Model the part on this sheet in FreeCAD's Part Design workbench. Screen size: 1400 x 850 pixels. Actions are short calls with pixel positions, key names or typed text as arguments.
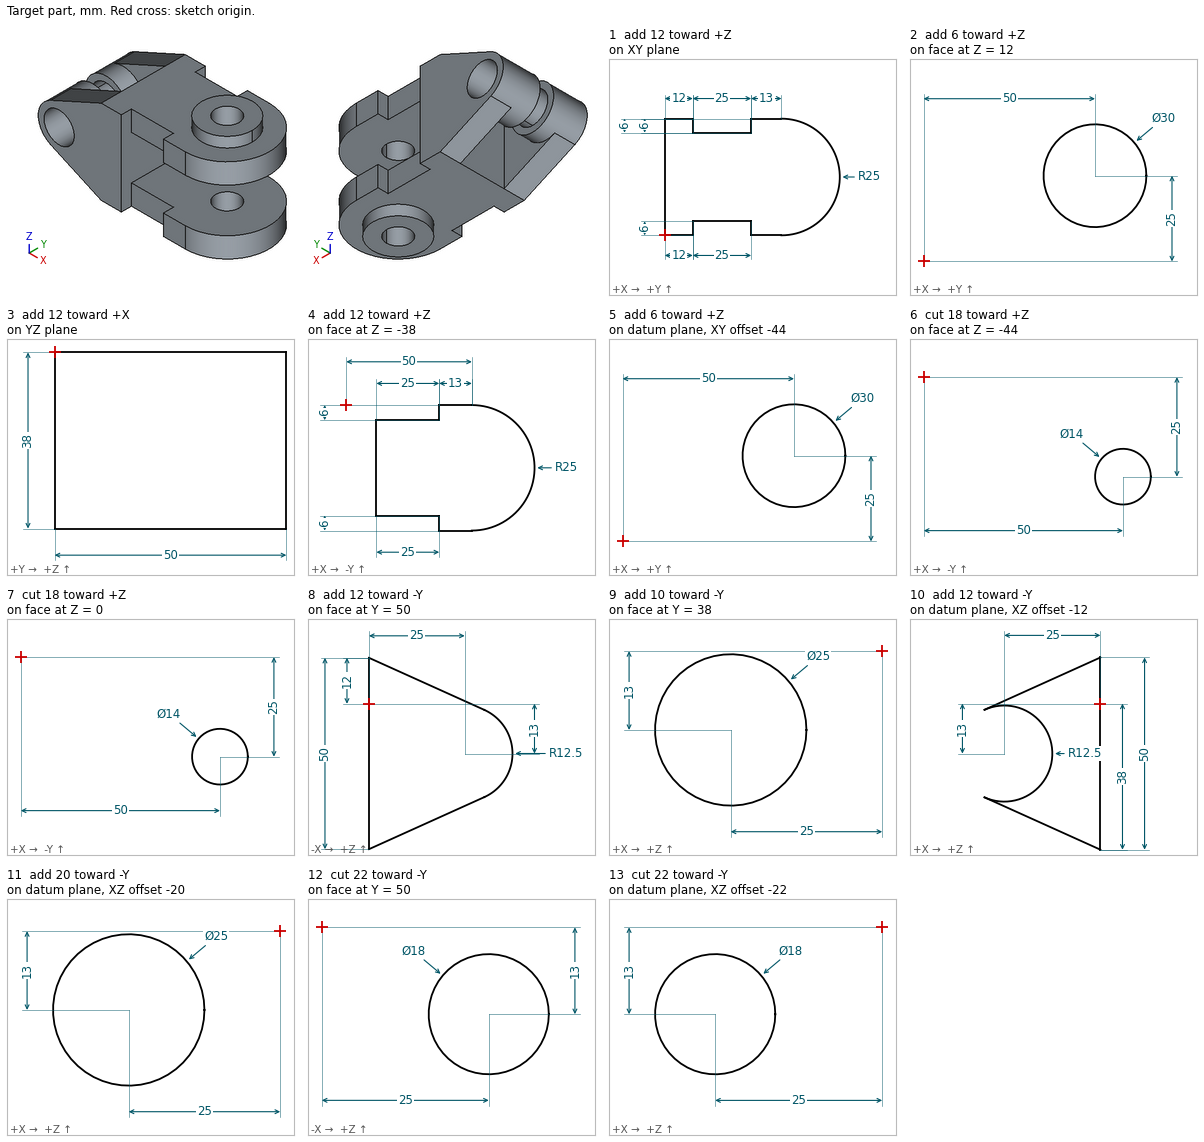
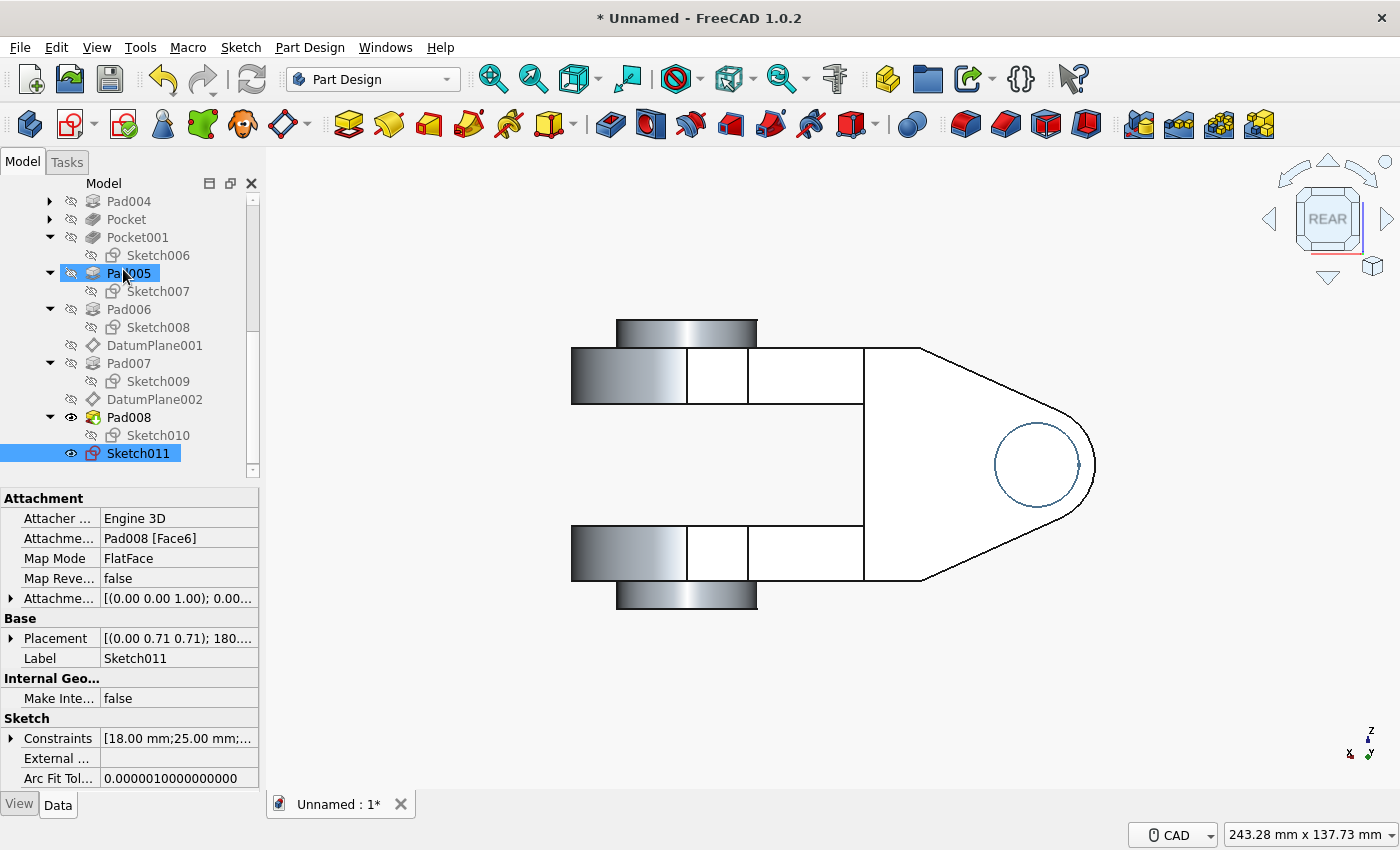
click(612, 124)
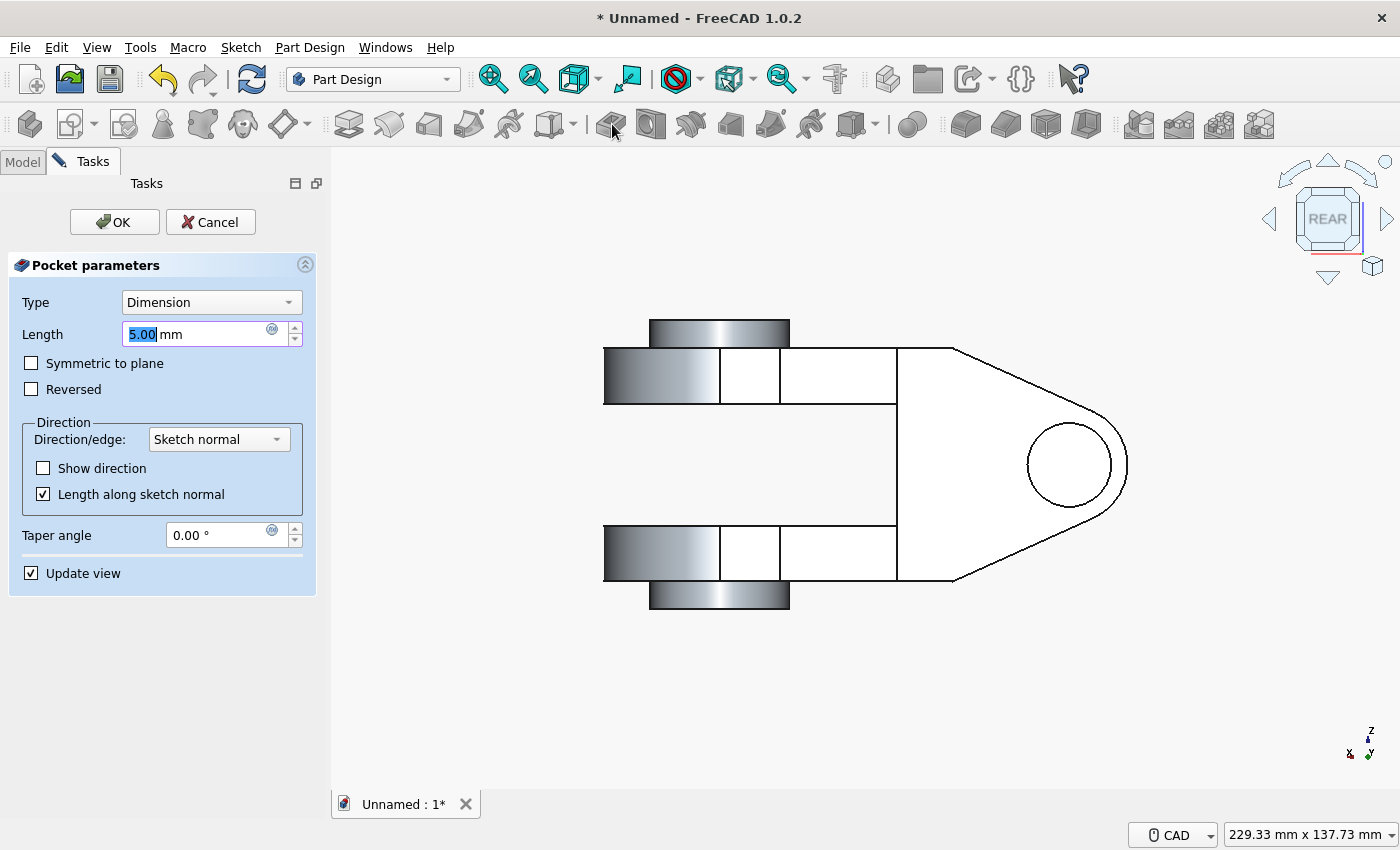
text(22)
key(Tab)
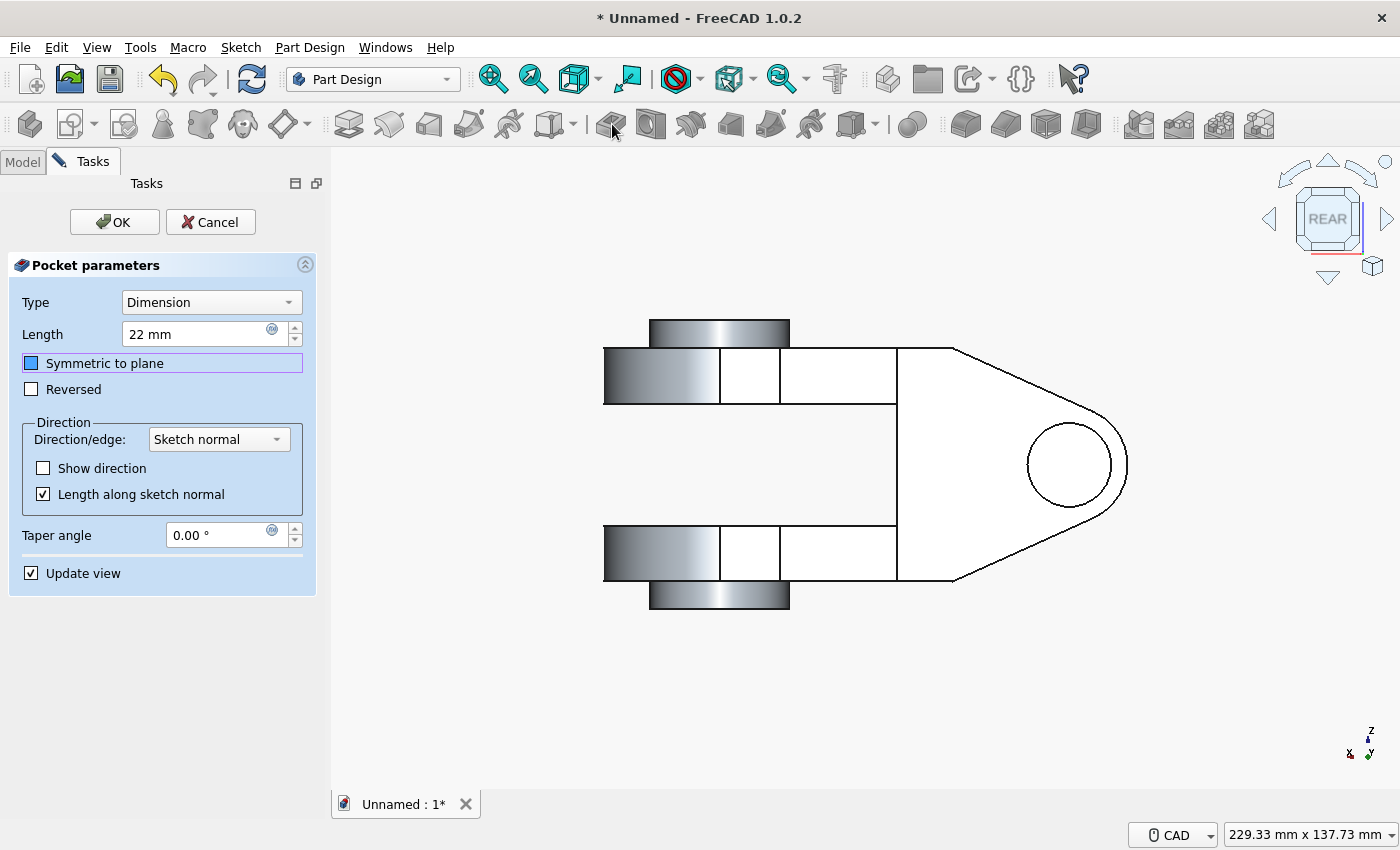
click(115, 222)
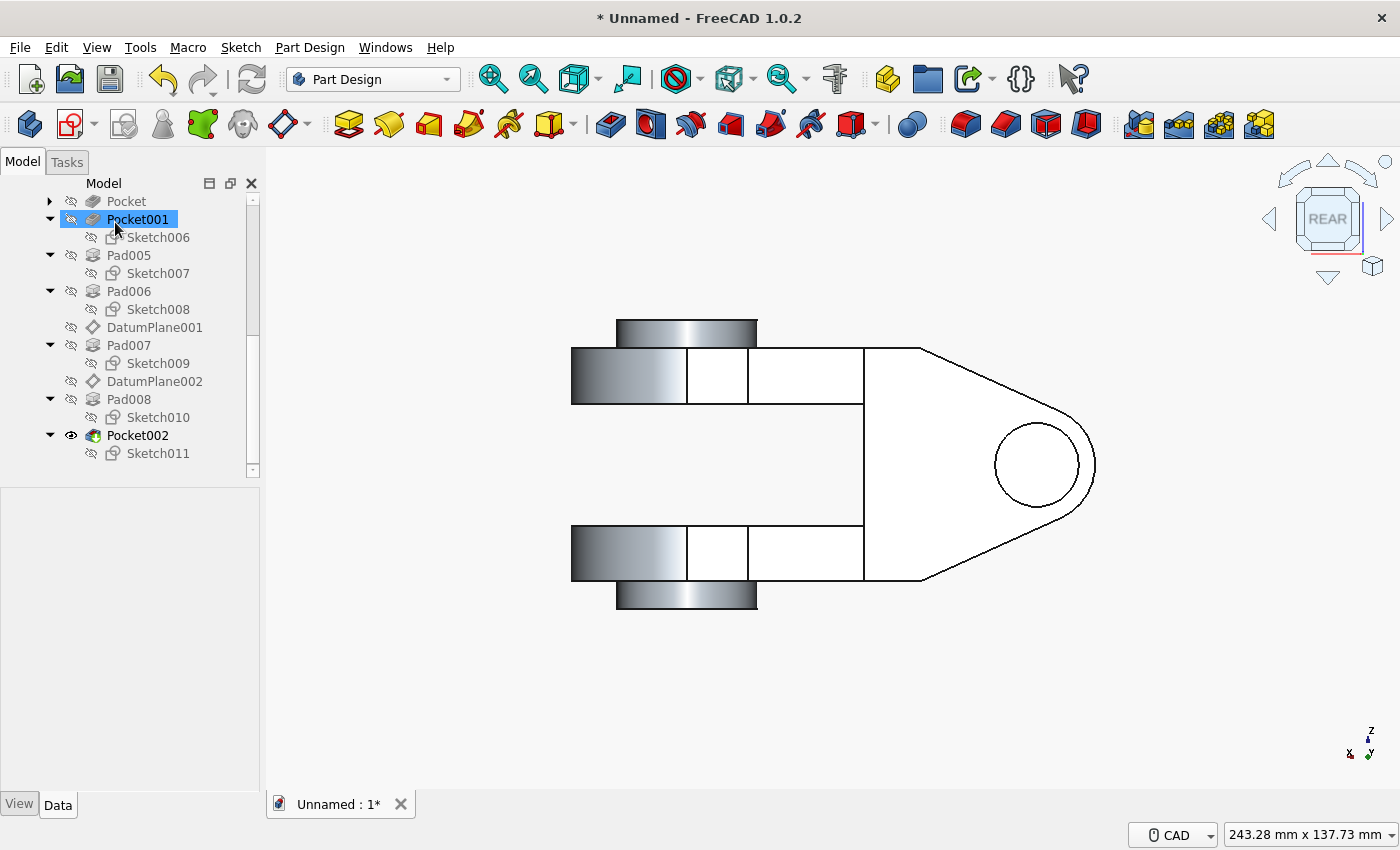
scroll(140, 323, down, 3)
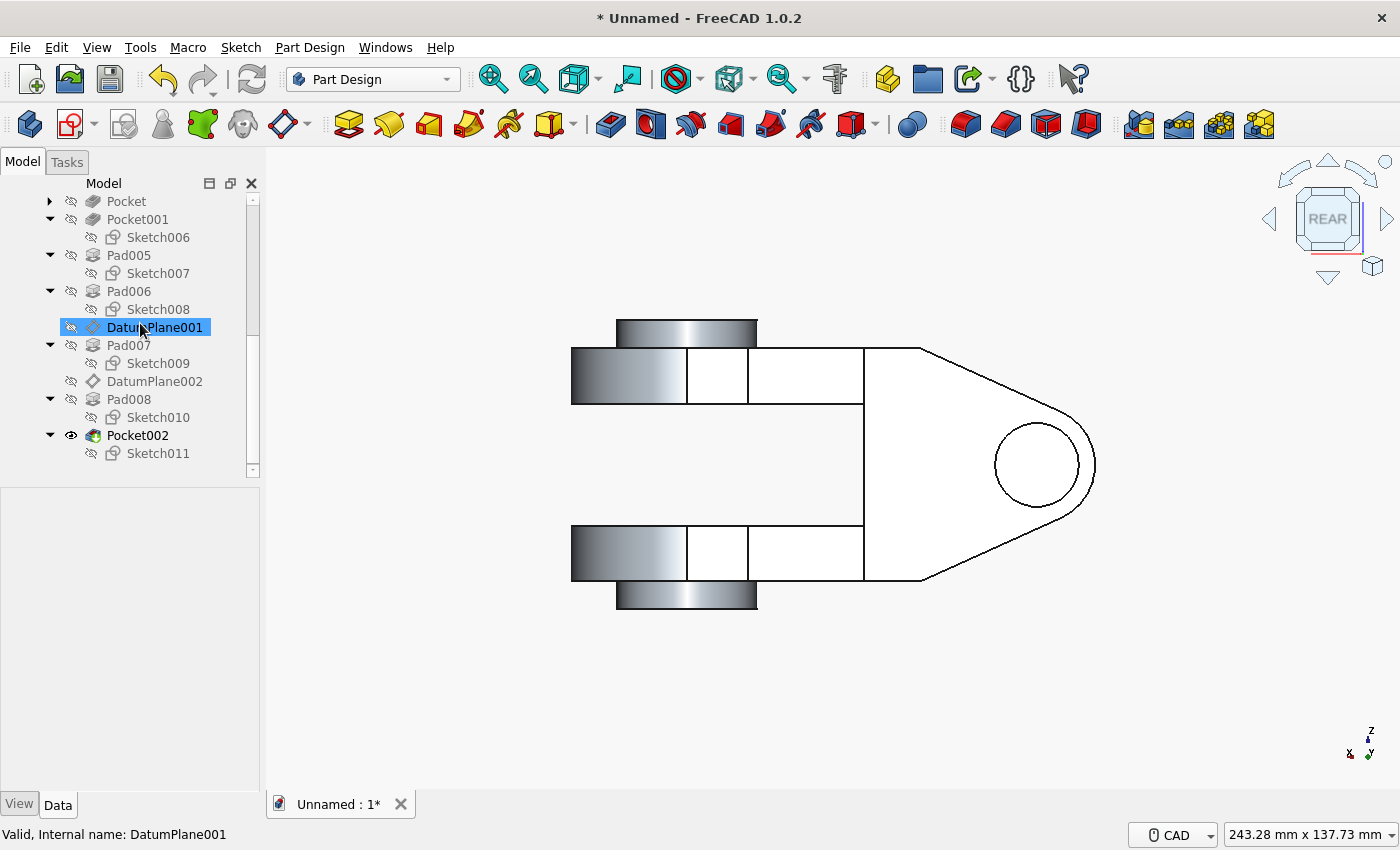
scroll(140, 323, up, 15)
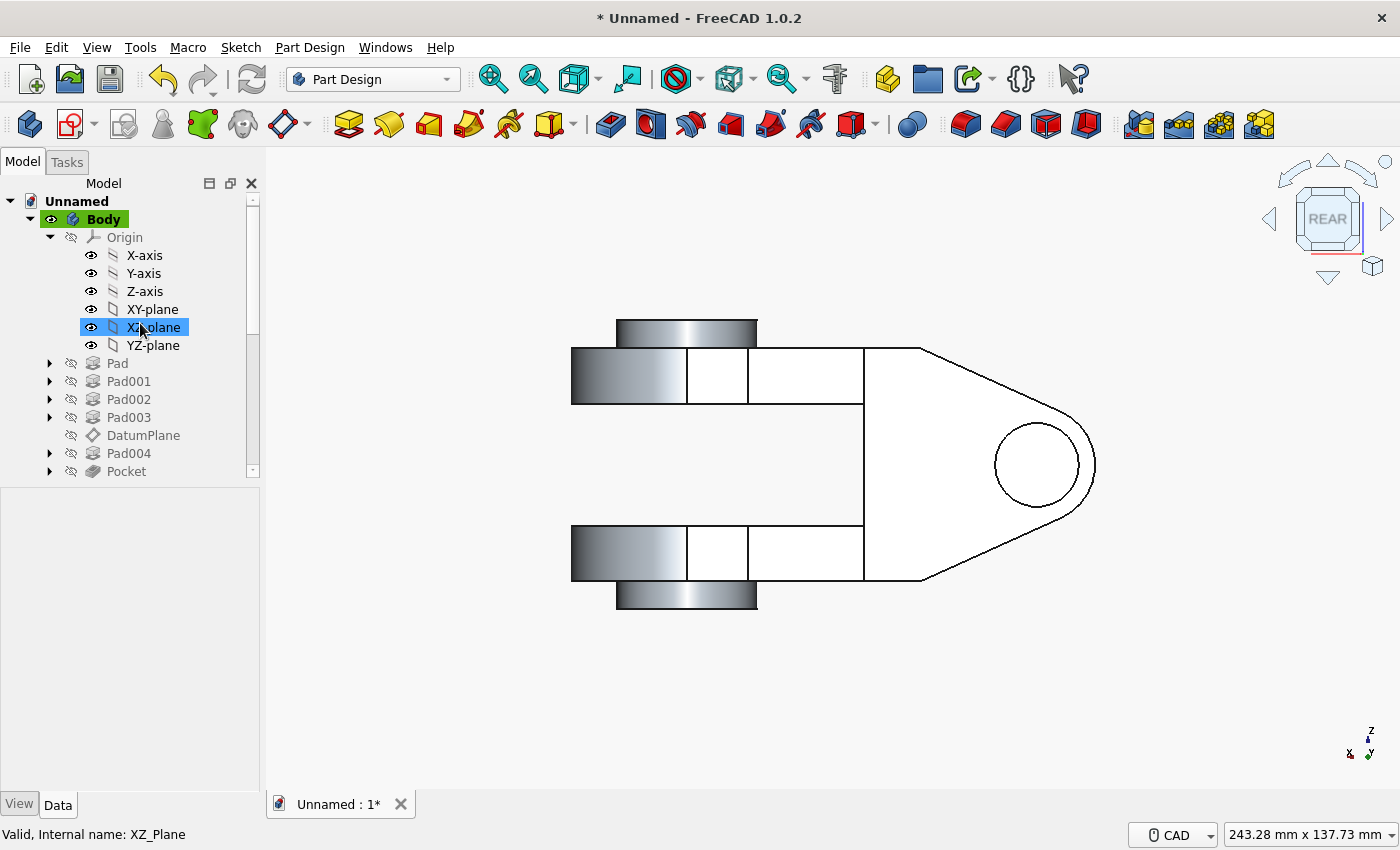
click(136, 327)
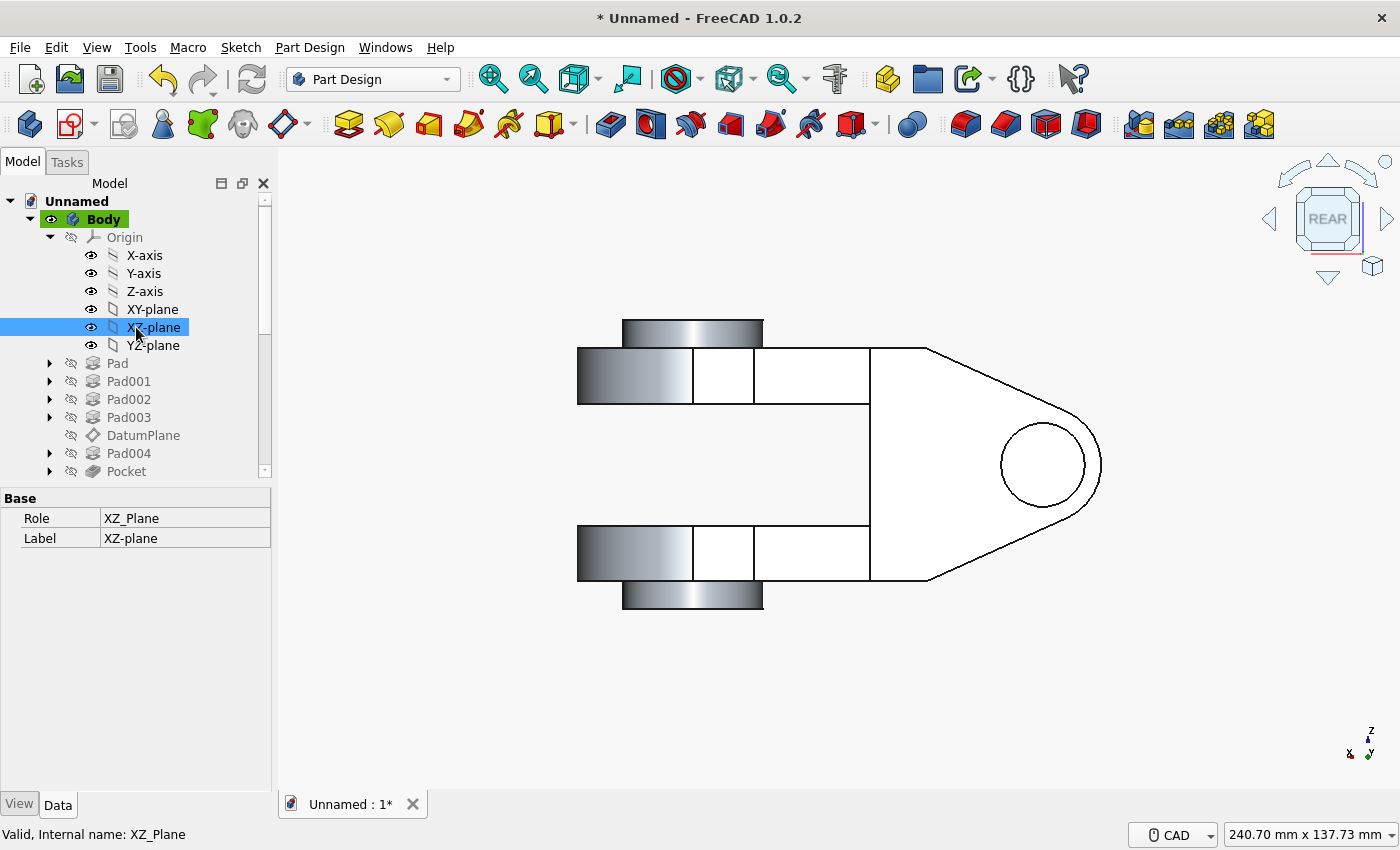
click(284, 124)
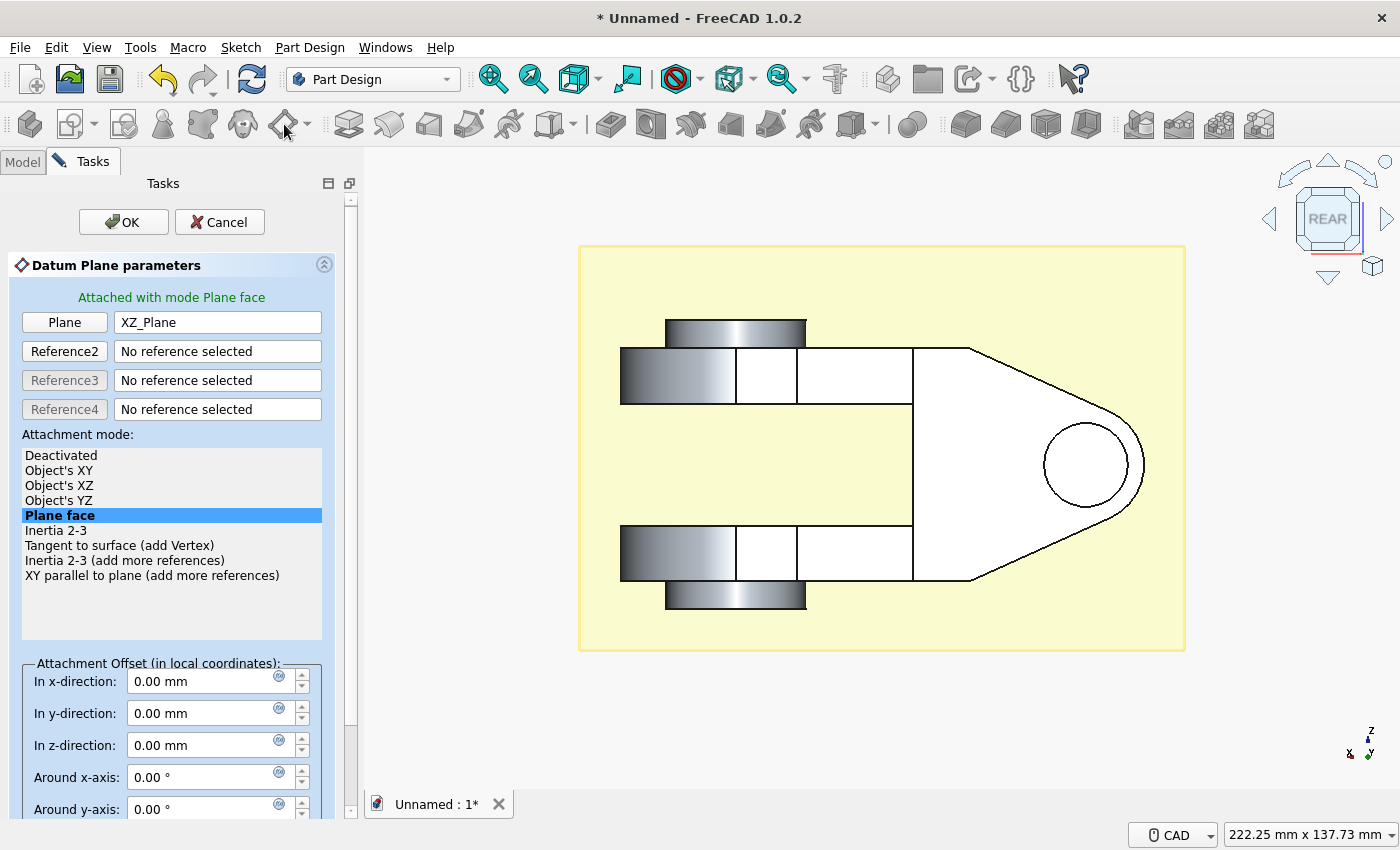
triple_click(210, 745)